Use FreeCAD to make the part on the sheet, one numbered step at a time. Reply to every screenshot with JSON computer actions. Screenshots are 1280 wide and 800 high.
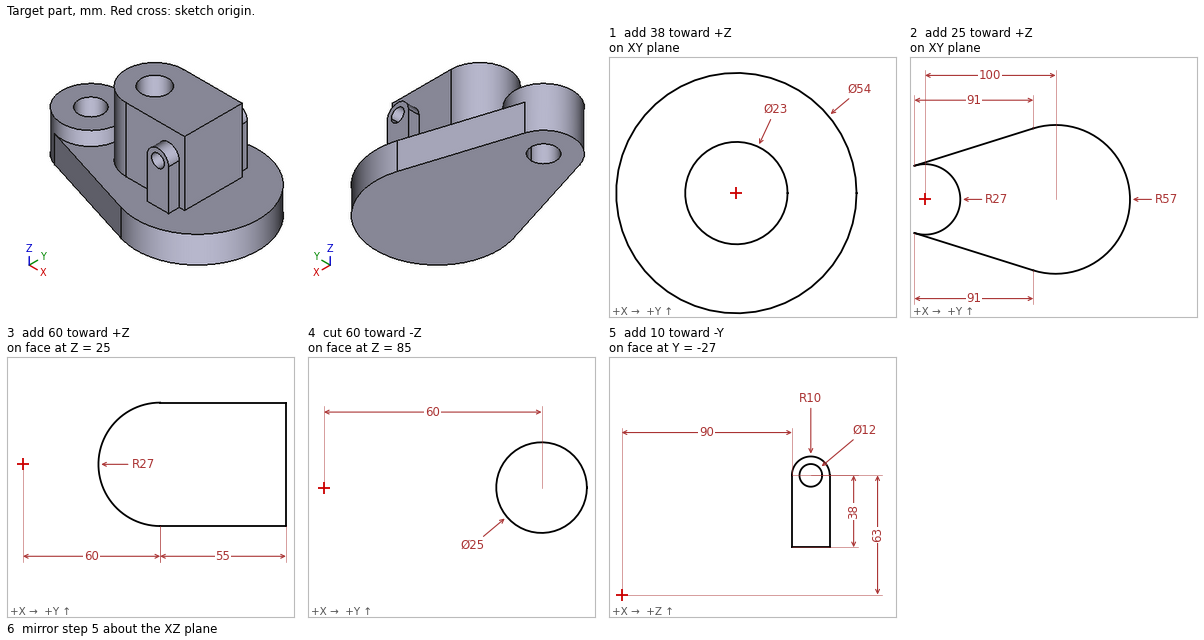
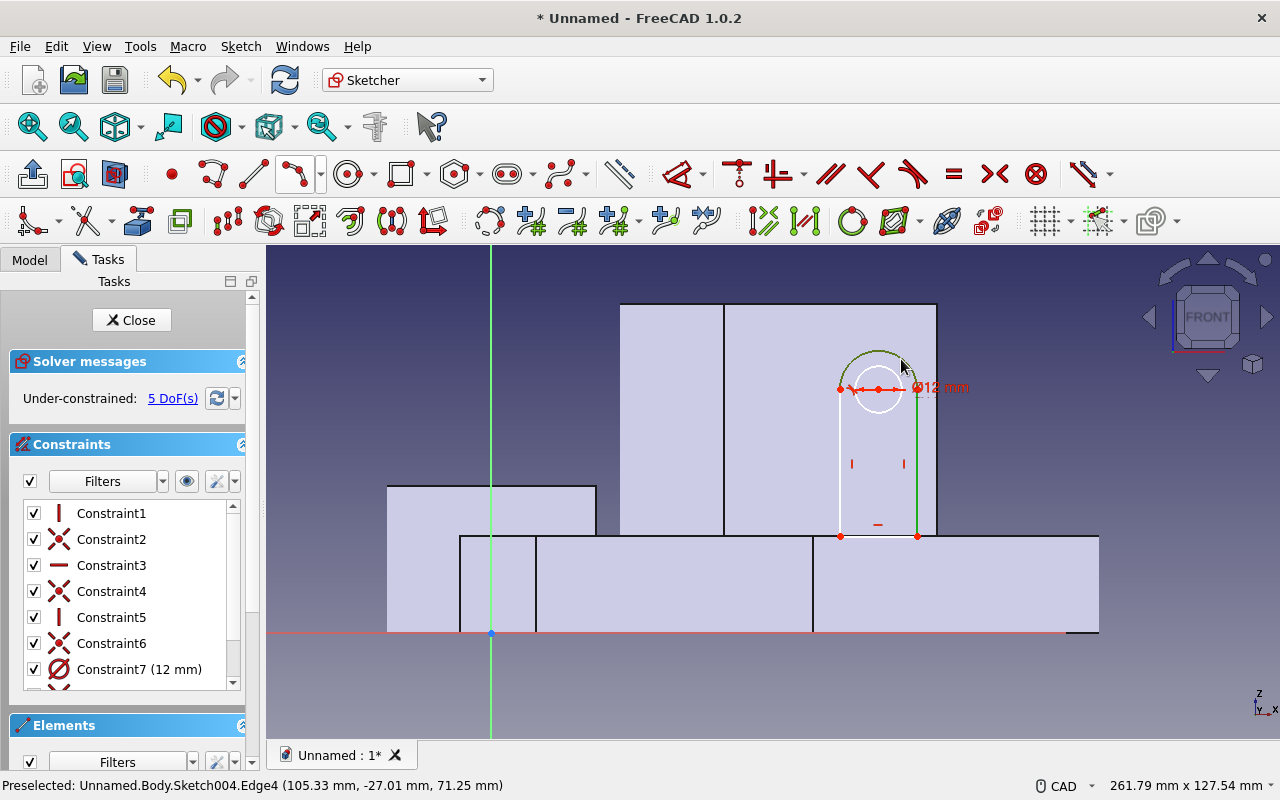
{"action": "key", "text": "t"}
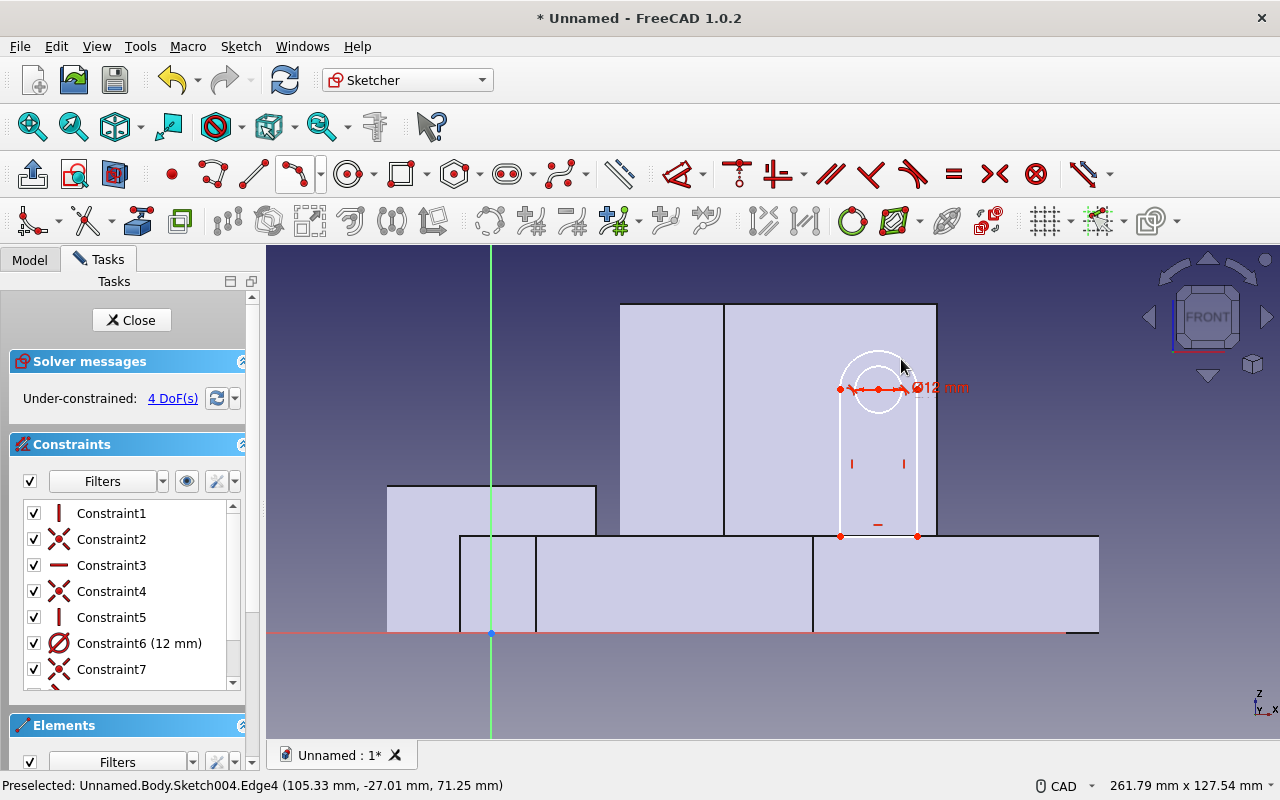
{"action": "left_click", "coordinate": [676, 174]}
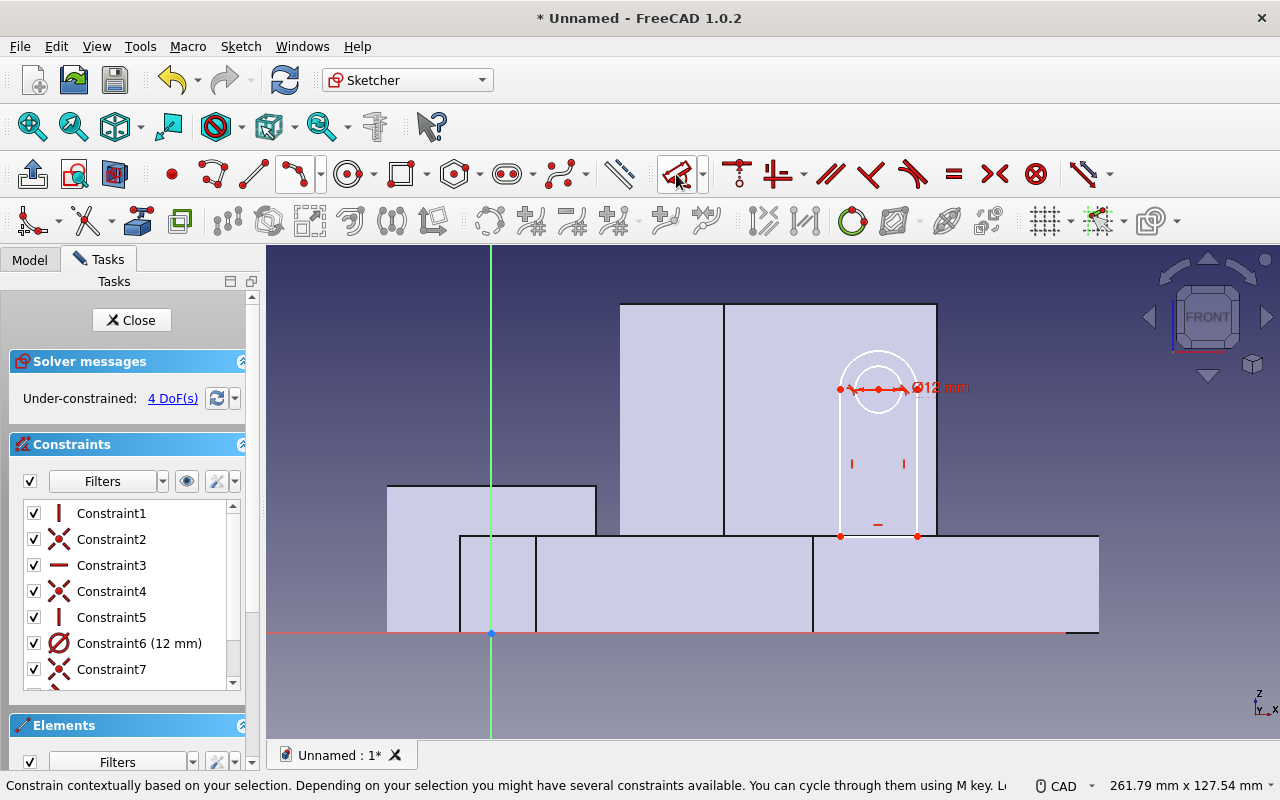
{"action": "left_click", "coordinate": [901, 358]}
{"action": "left_click", "coordinate": [920, 332]}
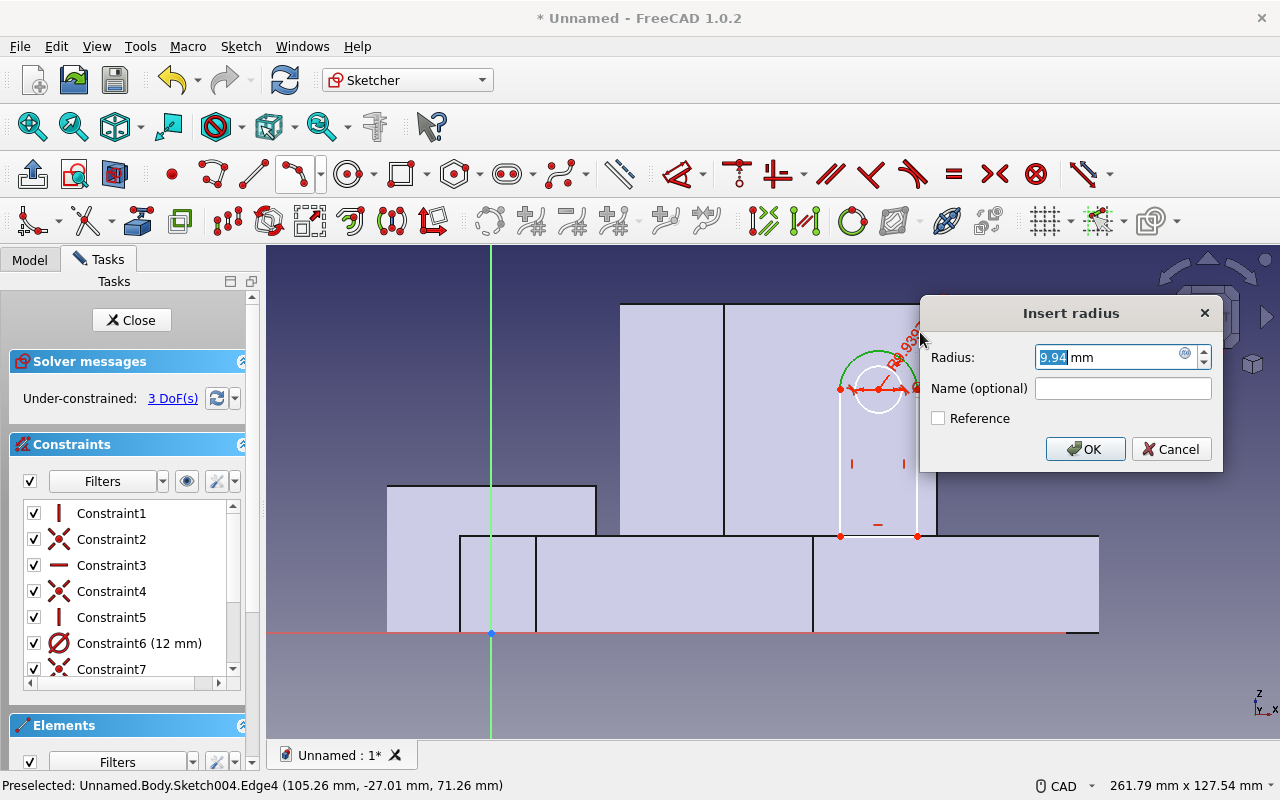
{"action": "type", "text": "10"}
{"action": "key", "text": "Return"}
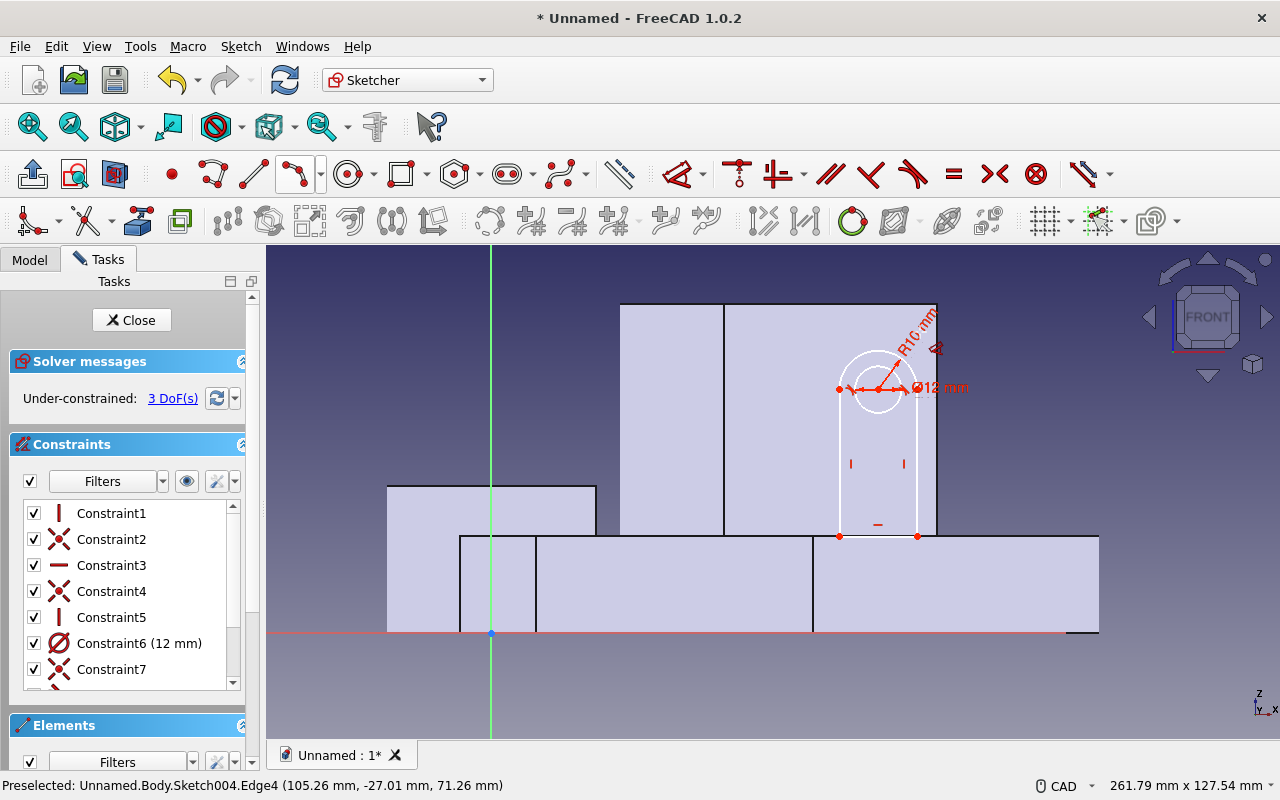
{"action": "left_click", "coordinate": [840, 434]}
{"action": "left_click", "coordinate": [874, 463]}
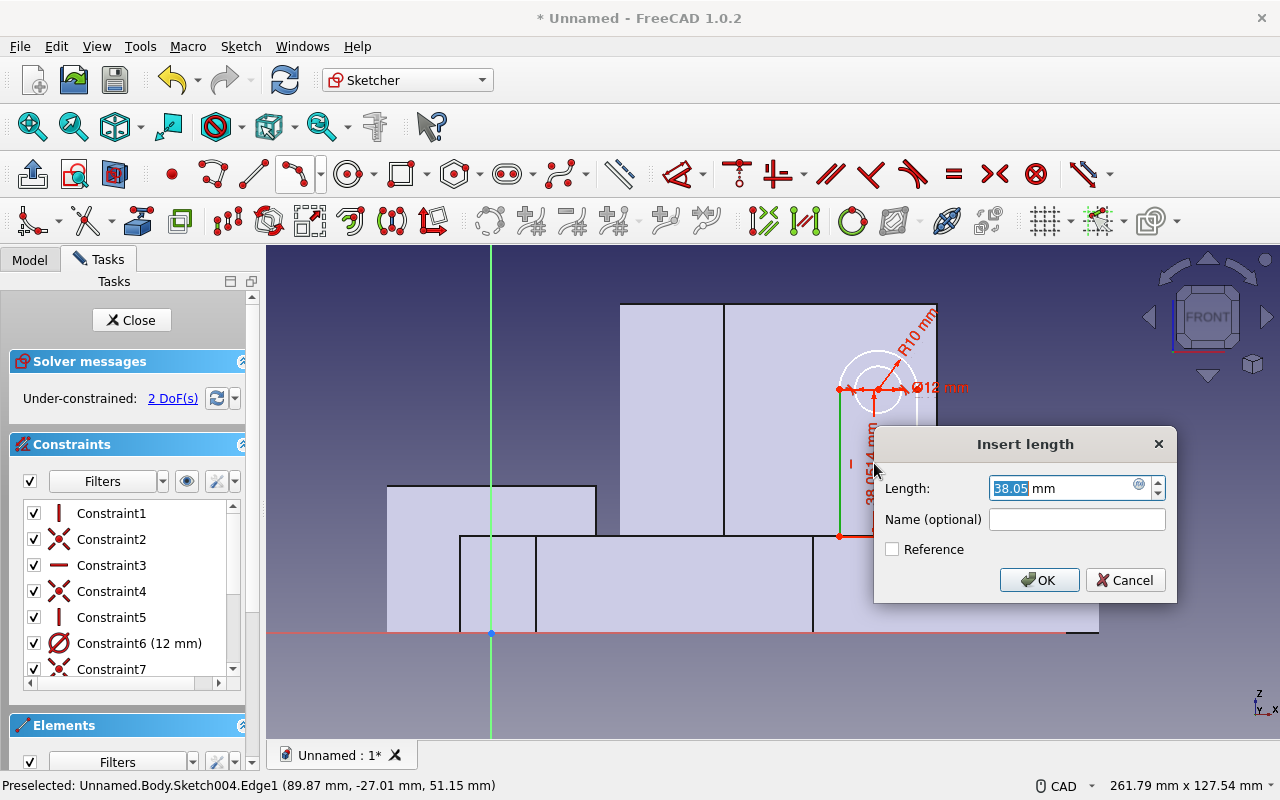
{"action": "type", "text": "38"}
{"action": "key", "text": "Return"}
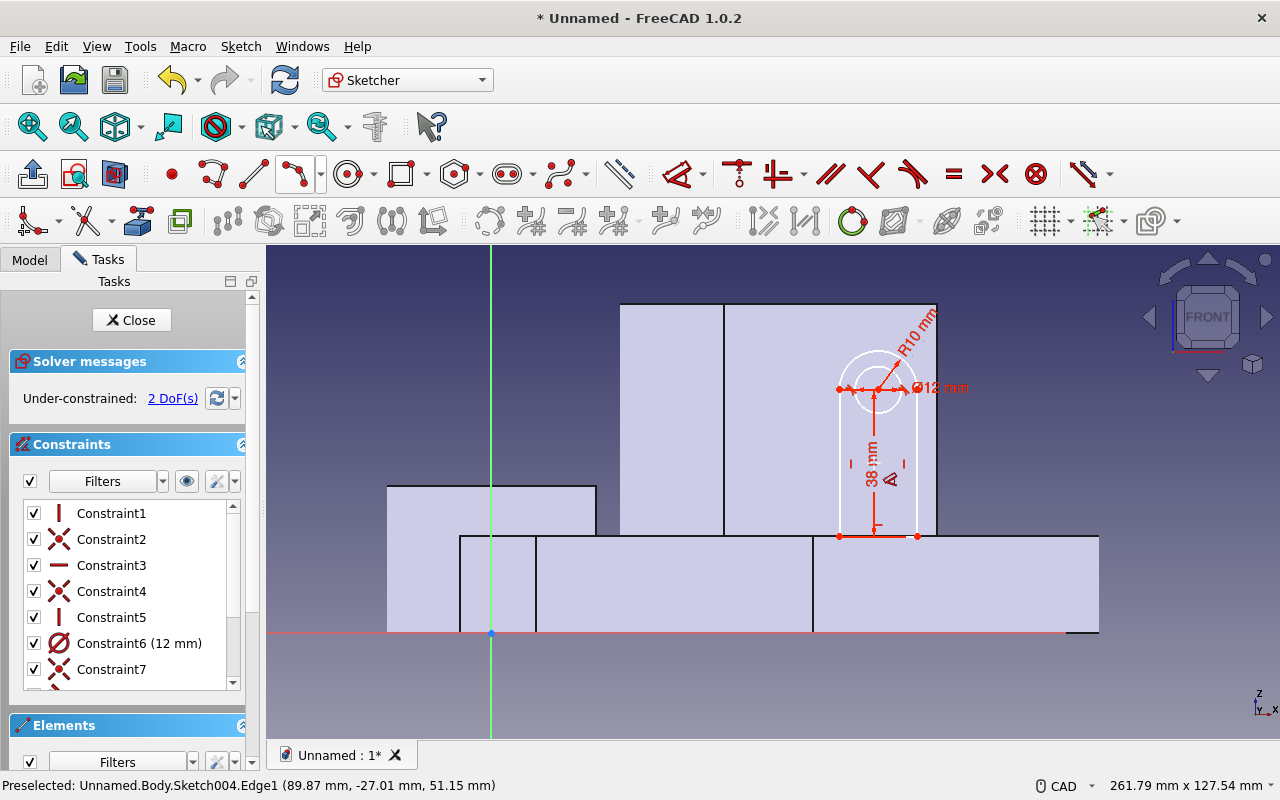
{"action": "left_click", "coordinate": [878, 390]}
{"action": "left_click", "coordinate": [457, 511]}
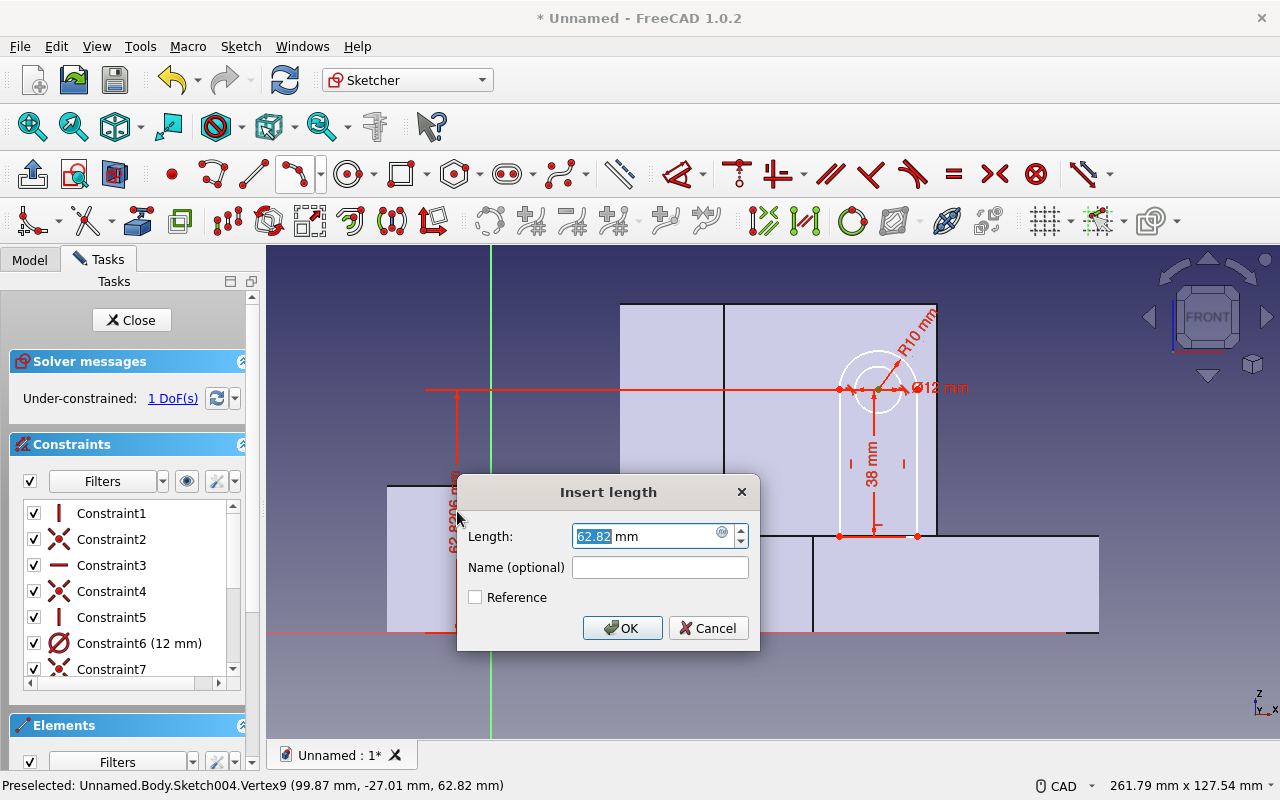
{"action": "type", "text": "63"}
{"action": "key", "text": "Return"}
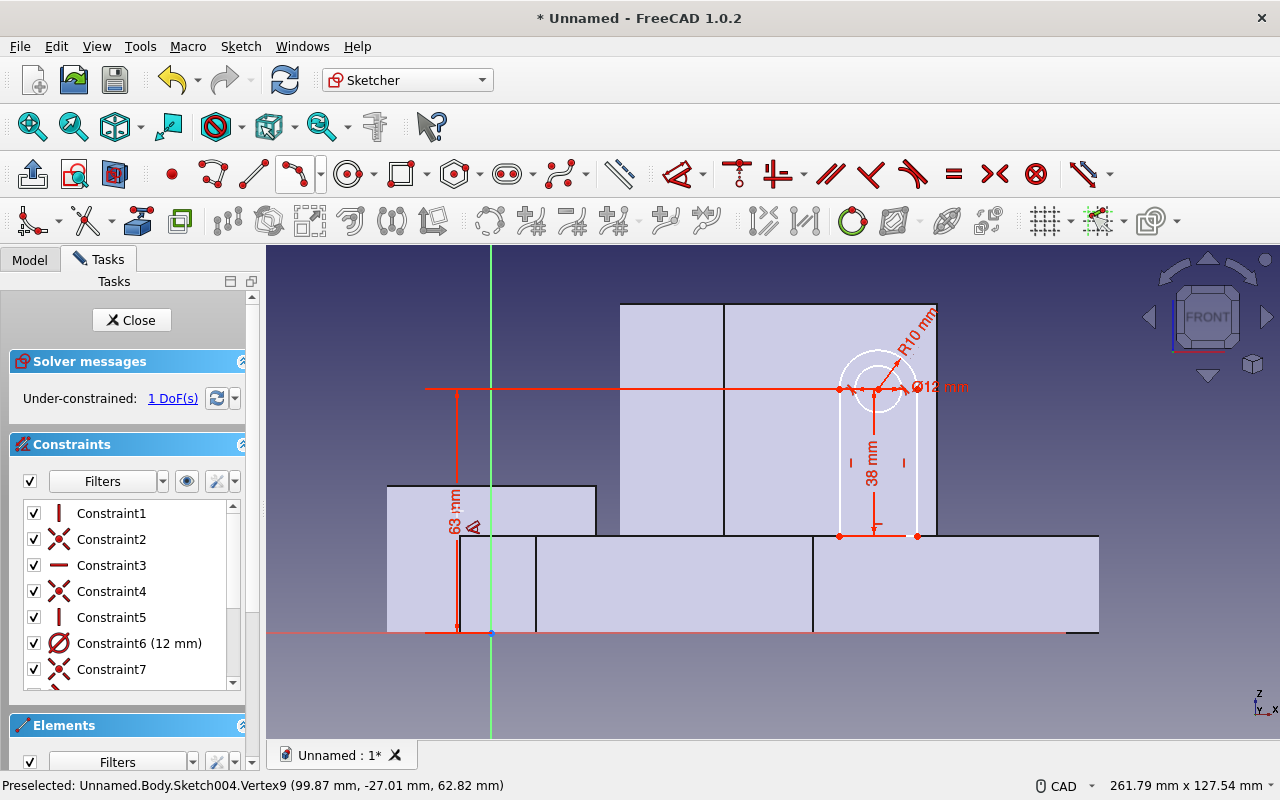
{"action": "left_click", "coordinate": [840, 389]}
{"action": "left_click", "coordinate": [665, 667]}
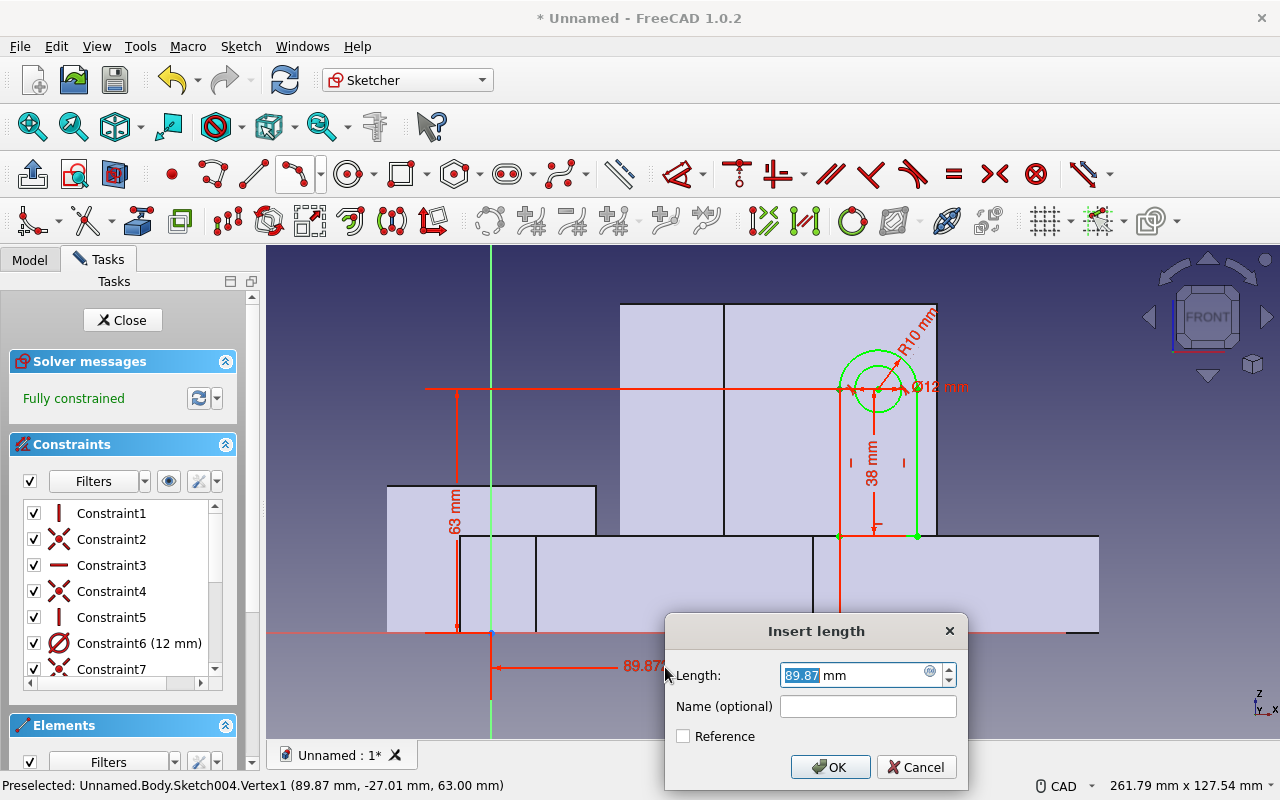
{"action": "type", "text": "90"}
{"action": "key", "text": "Return"}
{"action": "key", "text": "Escape"}